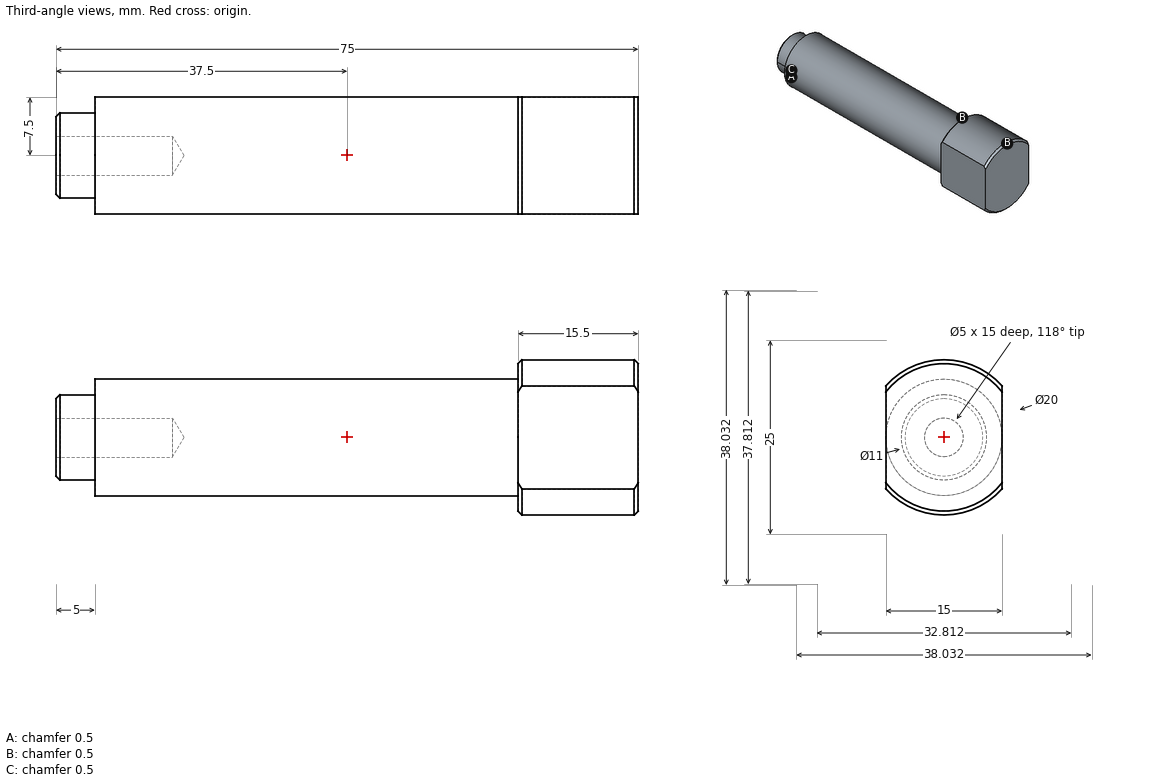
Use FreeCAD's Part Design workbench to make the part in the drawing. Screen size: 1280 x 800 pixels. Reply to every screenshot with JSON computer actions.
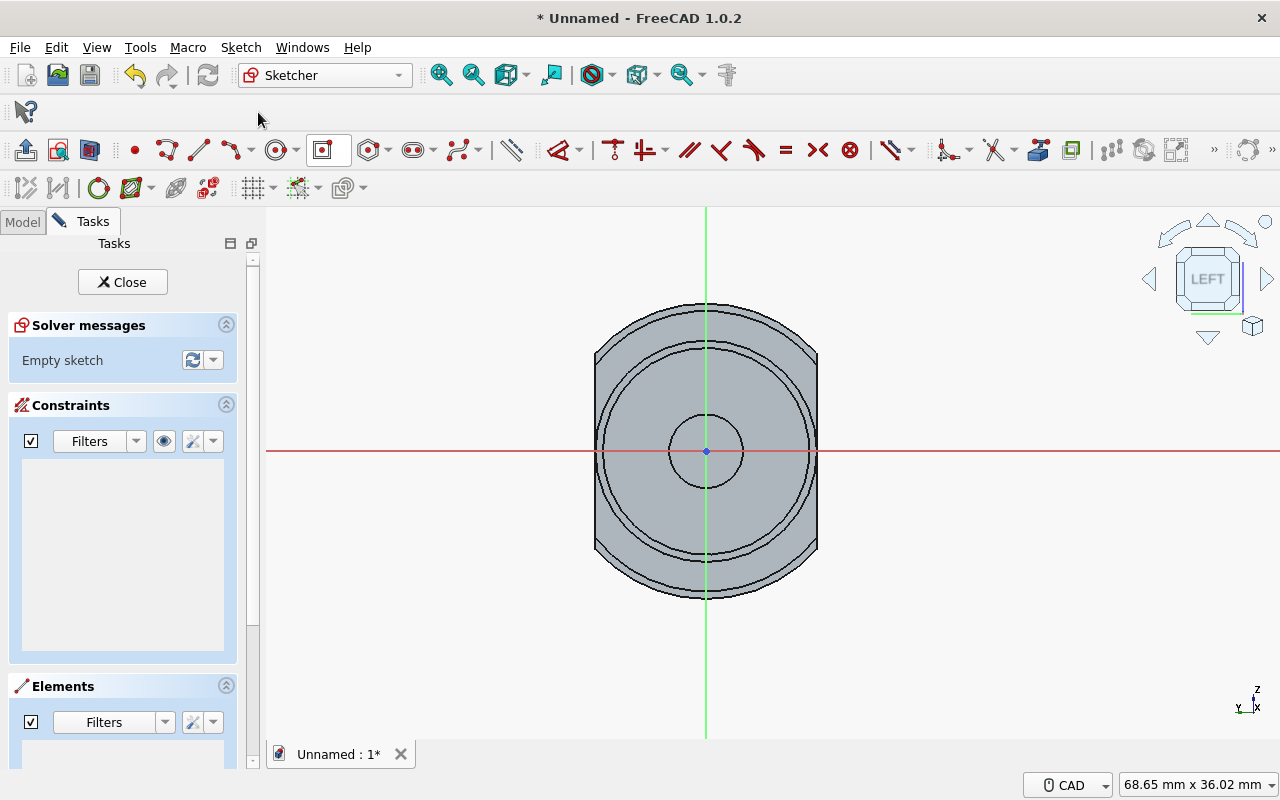
{"action": "scroll", "coordinate": [703, 499], "scroll_direction": "down", "scroll_amount": 3}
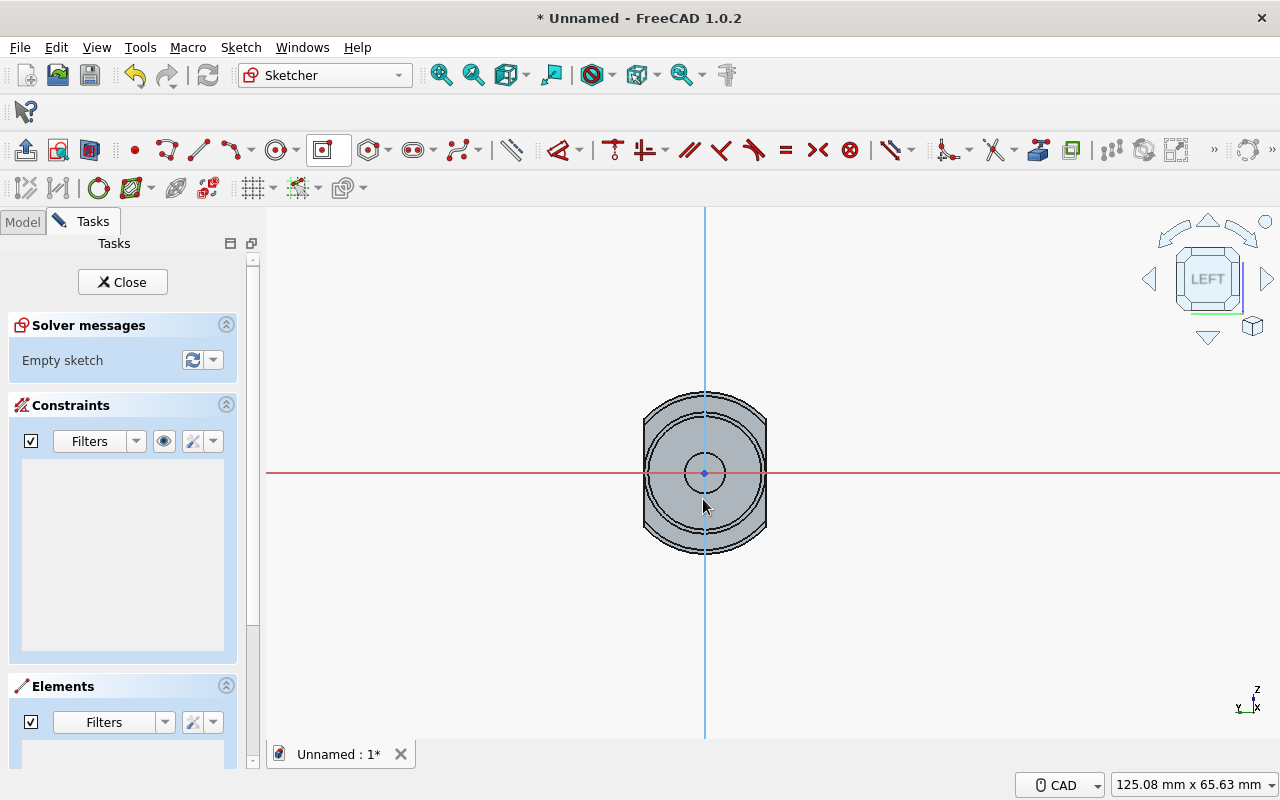
{"action": "key", "text": "g v"}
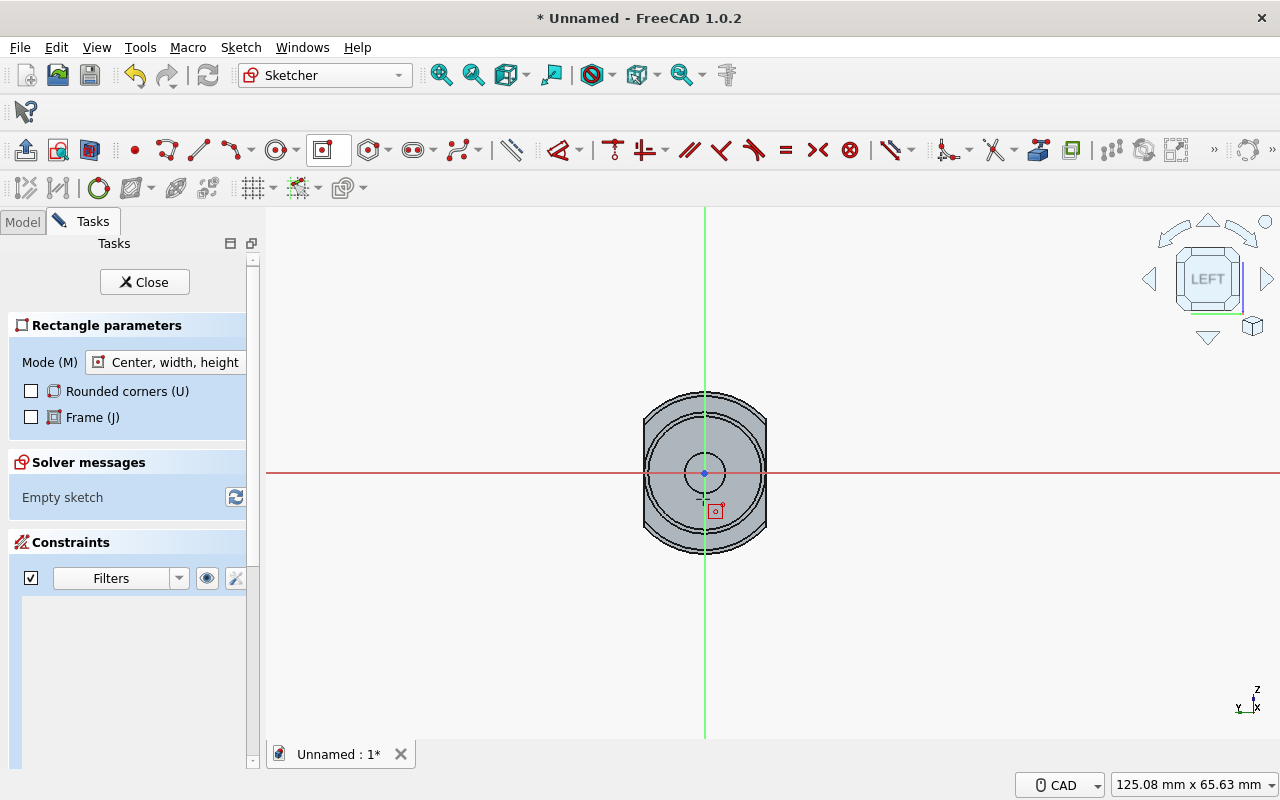
{"action": "left_click", "coordinate": [705, 473]}
{"action": "left_click", "coordinate": [838, 320]}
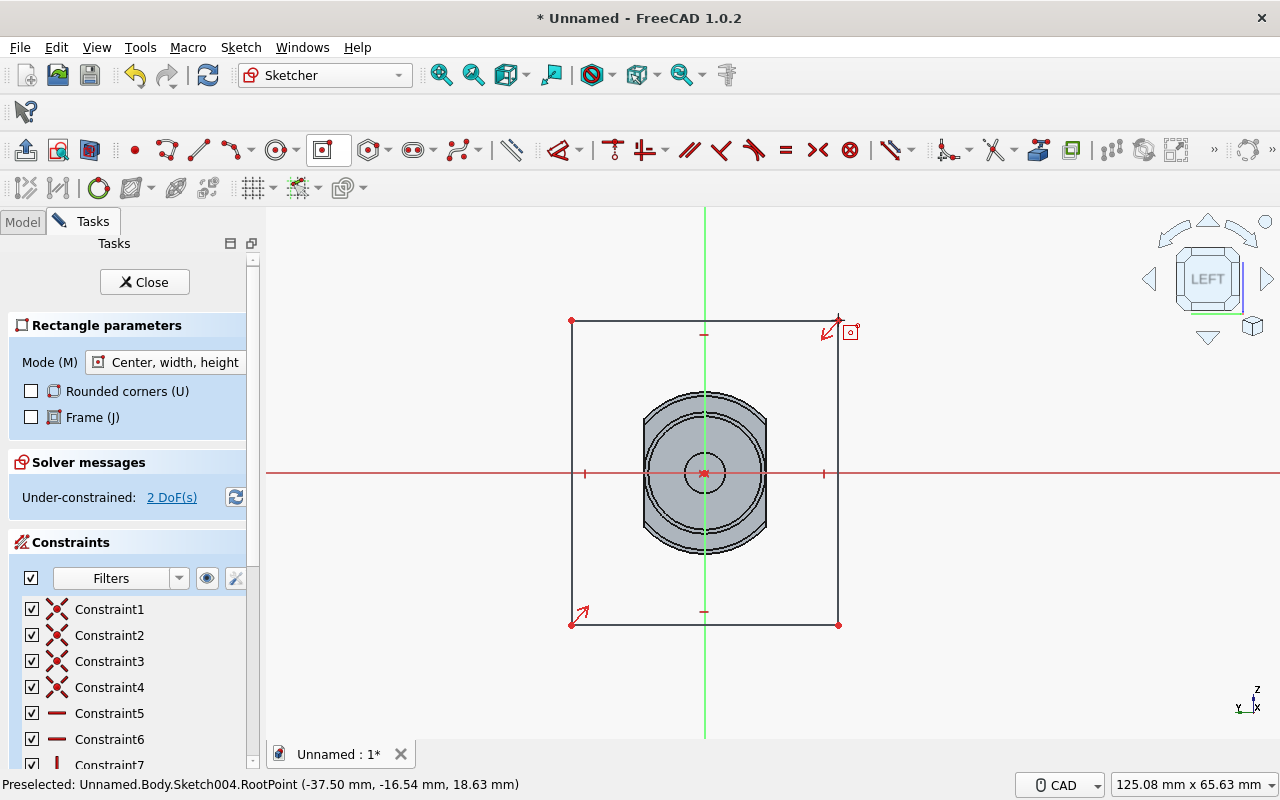
{"action": "left_click", "coordinate": [276, 150]}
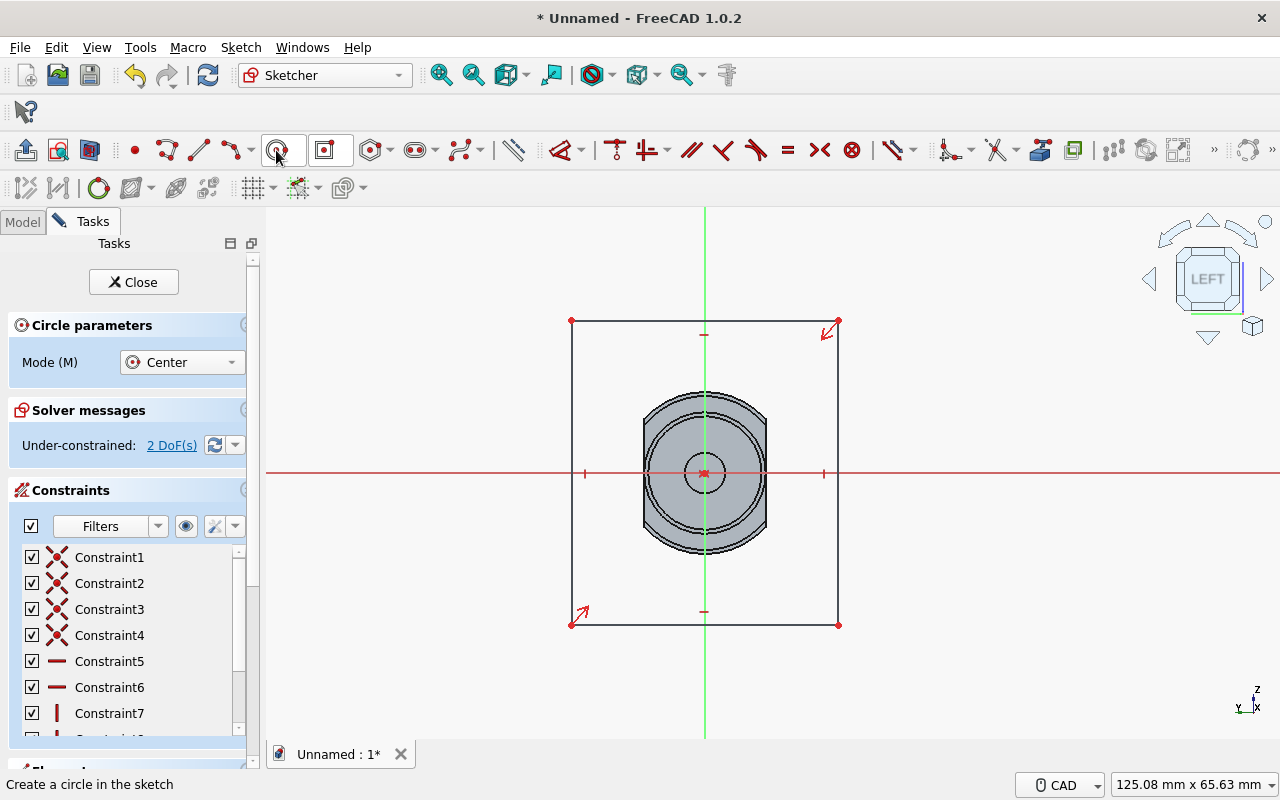
{"action": "left_click", "coordinate": [705, 473]}
{"action": "left_click", "coordinate": [736, 442]}
{"action": "key", "text": "Escape"}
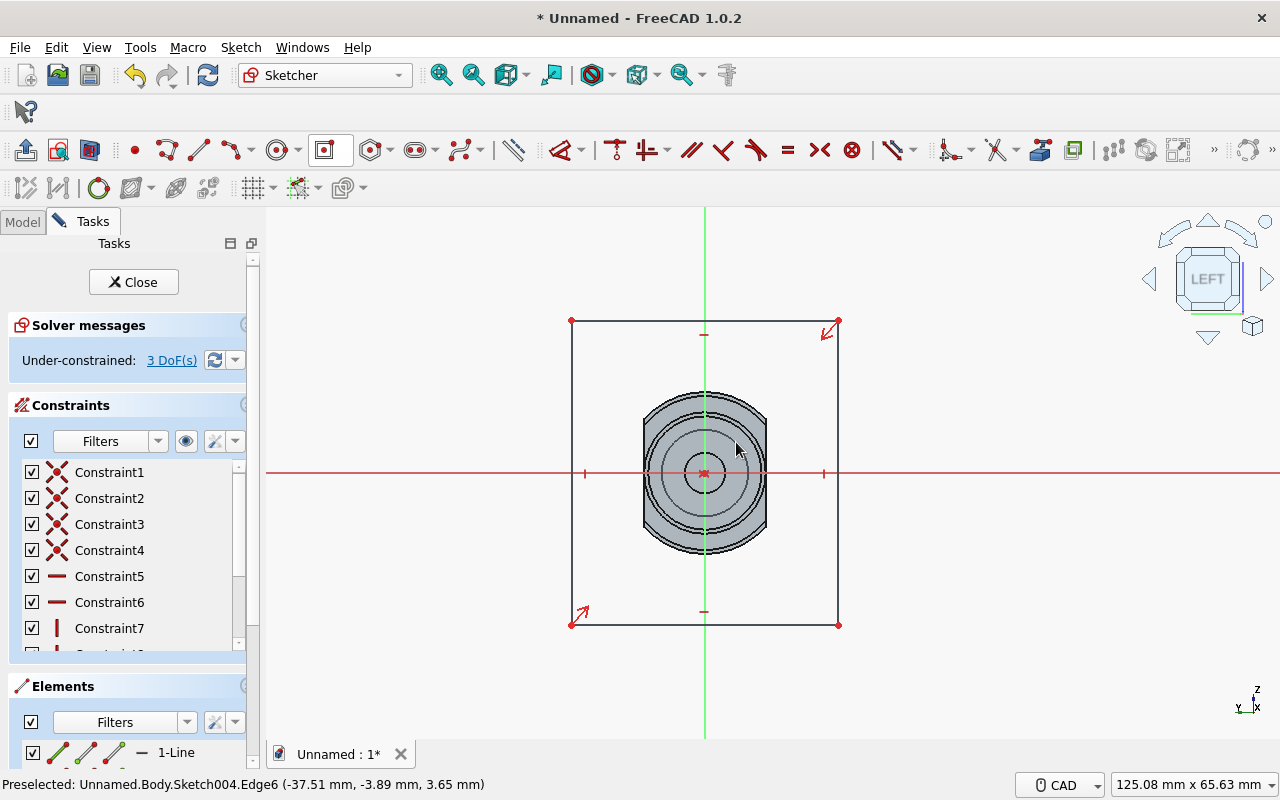
{"action": "left_click", "coordinate": [560, 150]}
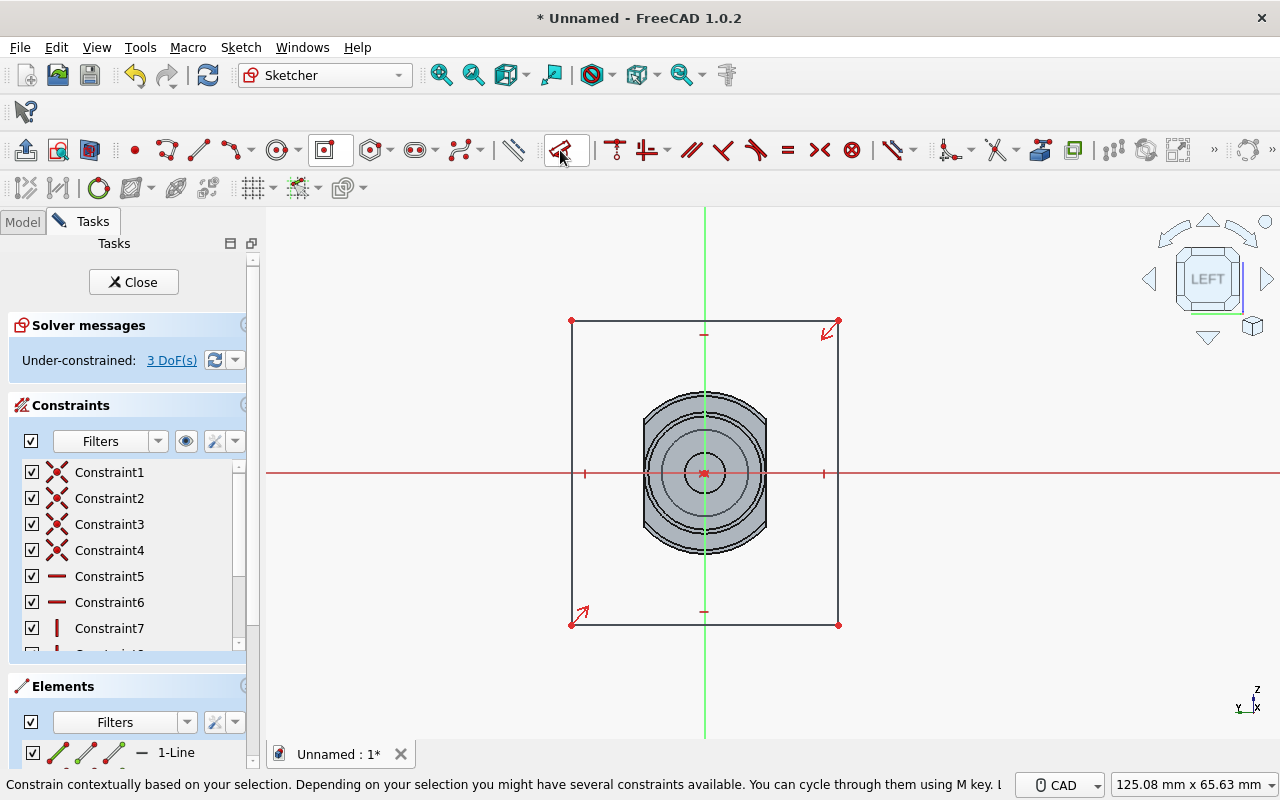
{"action": "left_click", "coordinate": [735, 442]}
{"action": "left_click", "coordinate": [757, 419]}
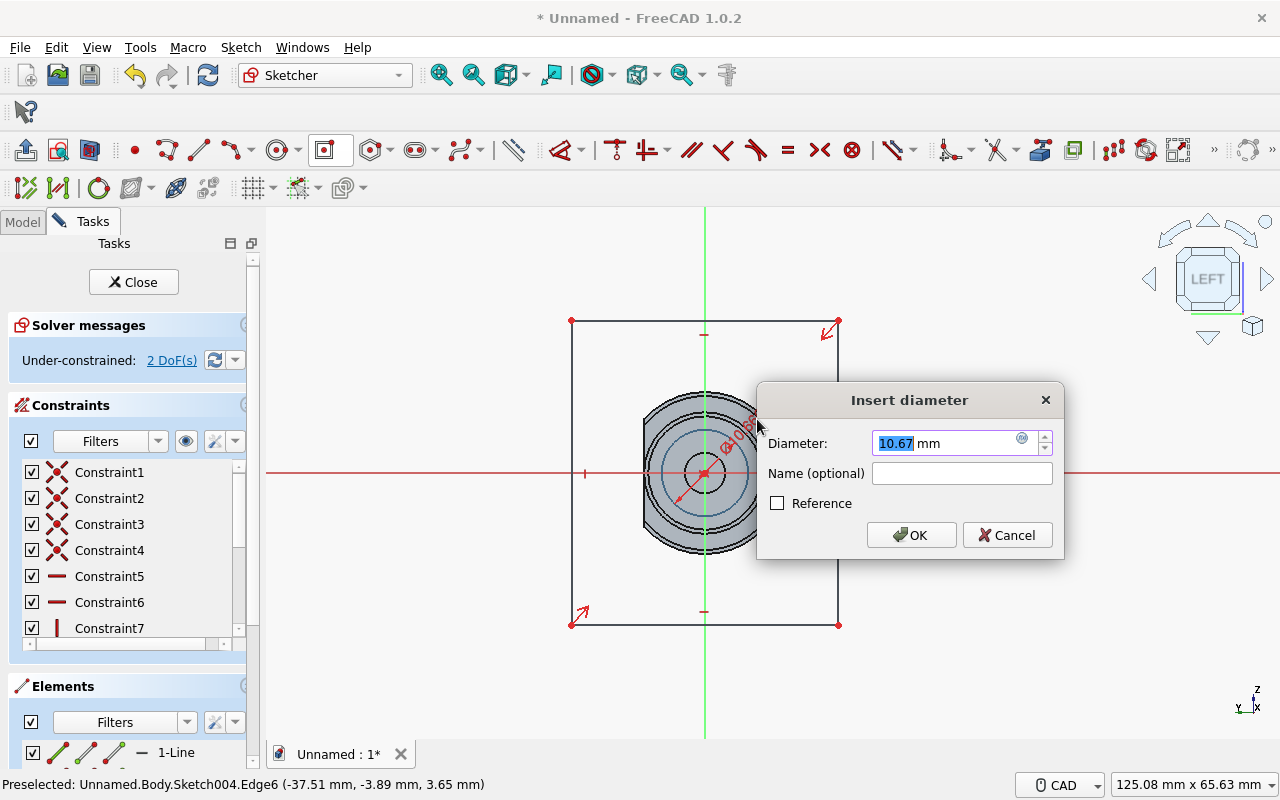
{"action": "type", "text": "11"}
{"action": "key", "text": "Return"}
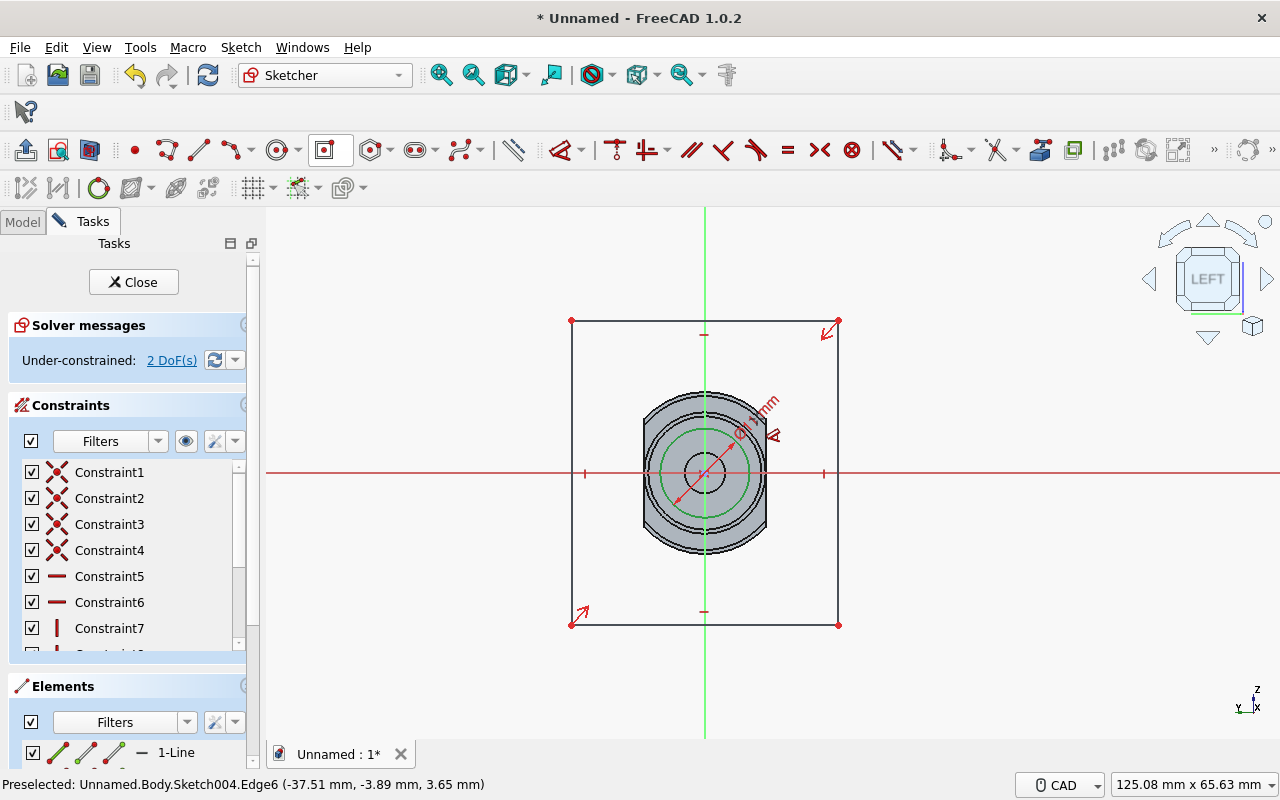
{"action": "left_click", "coordinate": [652, 625]}
{"action": "left_click", "coordinate": [644, 659]}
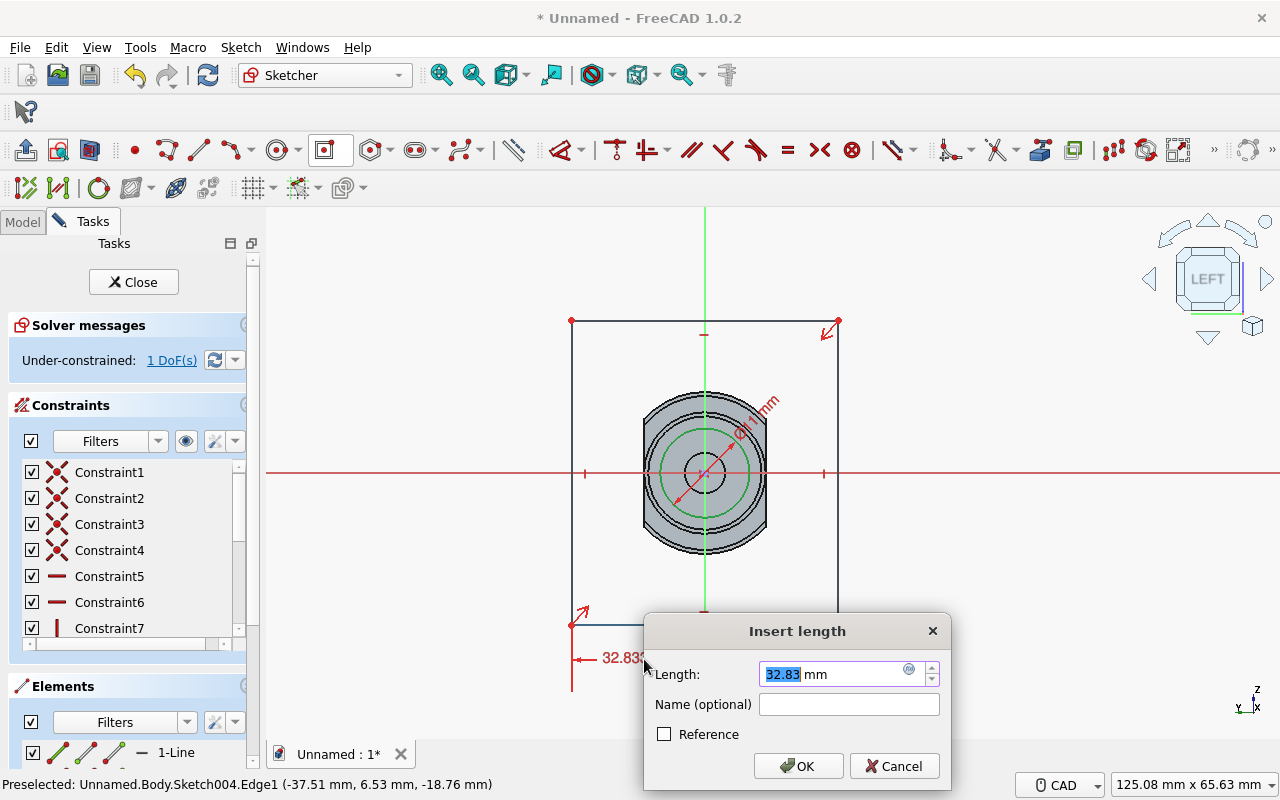
{"action": "type", "text": "32.812"}
{"action": "key", "text": "Return"}